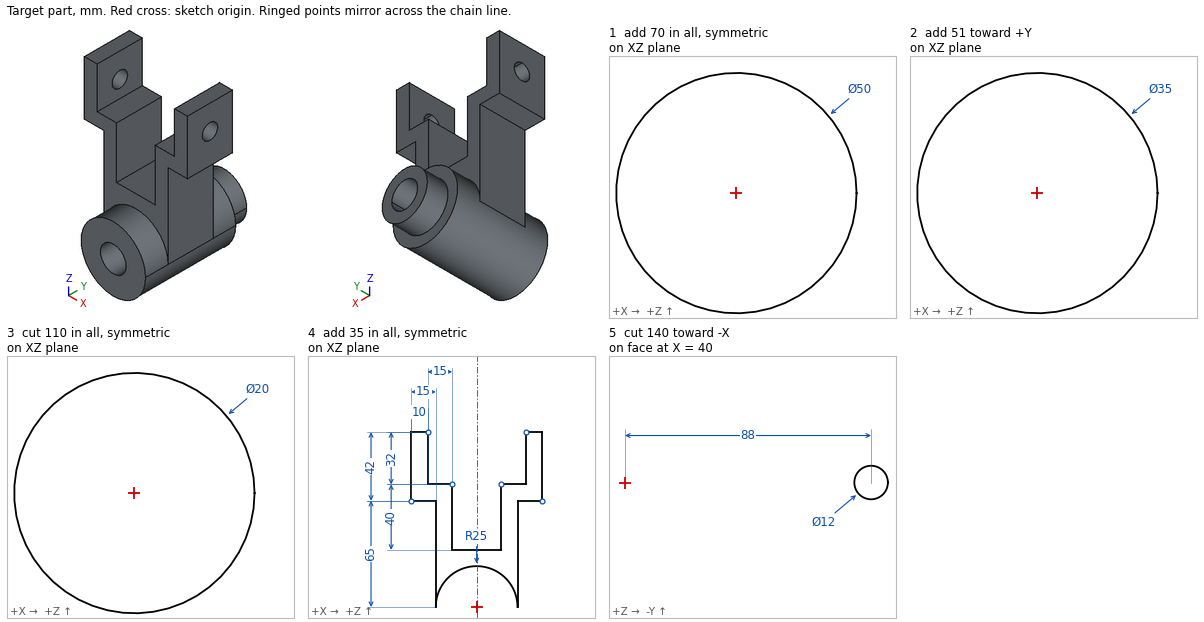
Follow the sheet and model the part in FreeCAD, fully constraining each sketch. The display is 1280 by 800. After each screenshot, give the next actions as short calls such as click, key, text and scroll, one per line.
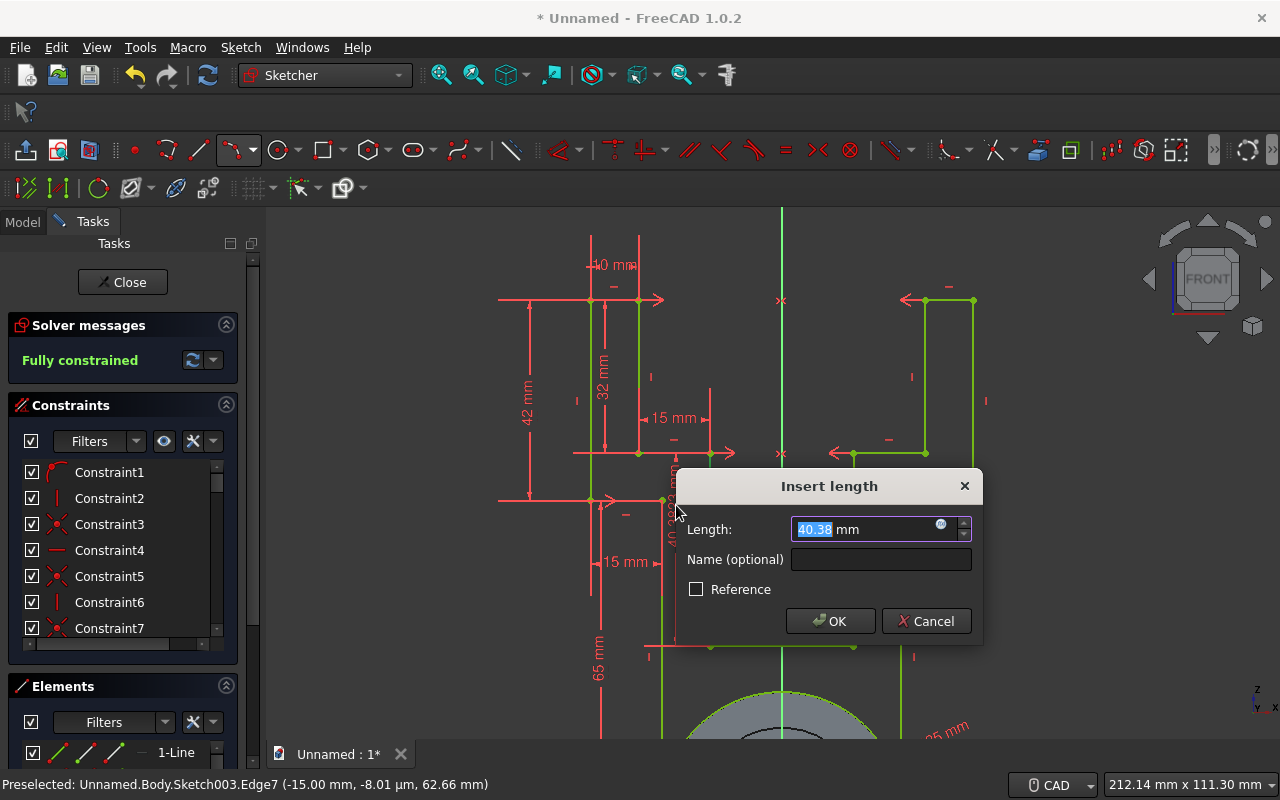
text(40)
key(Return)
key(Escape)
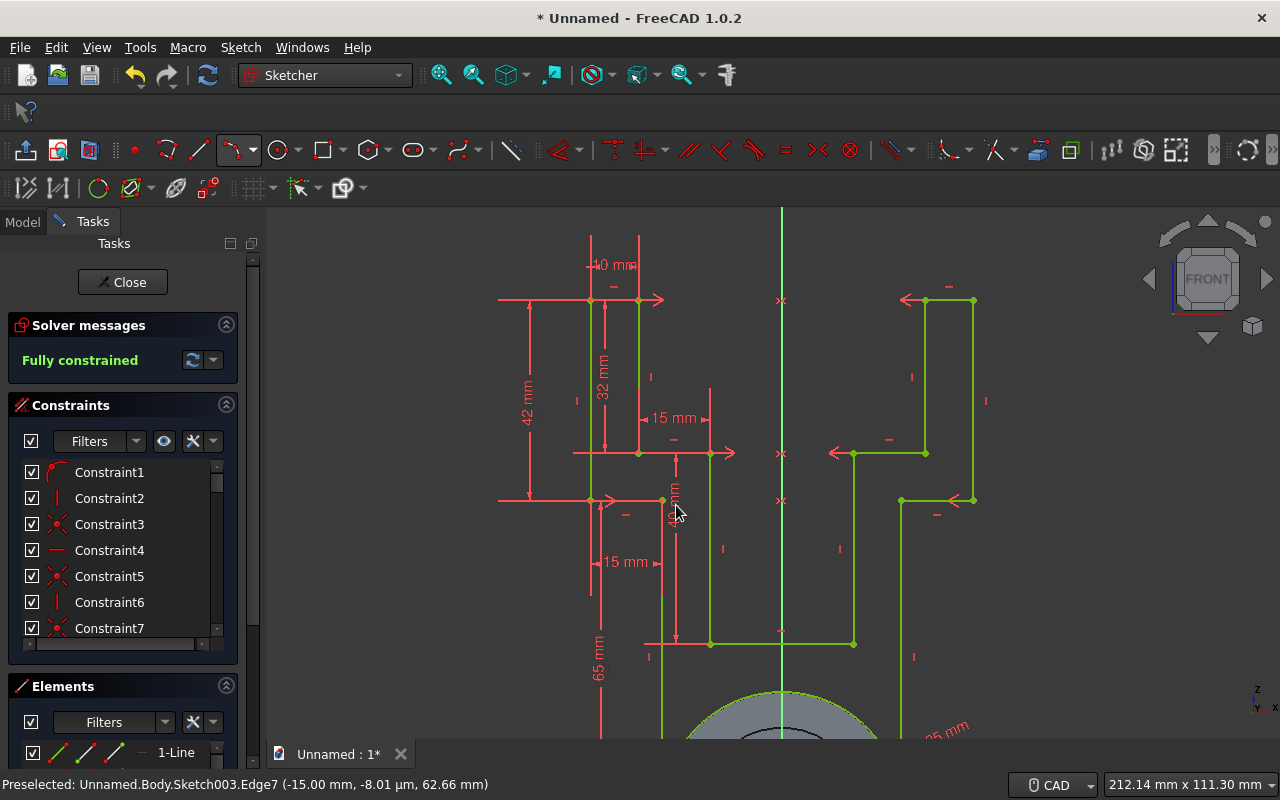
click(123, 282)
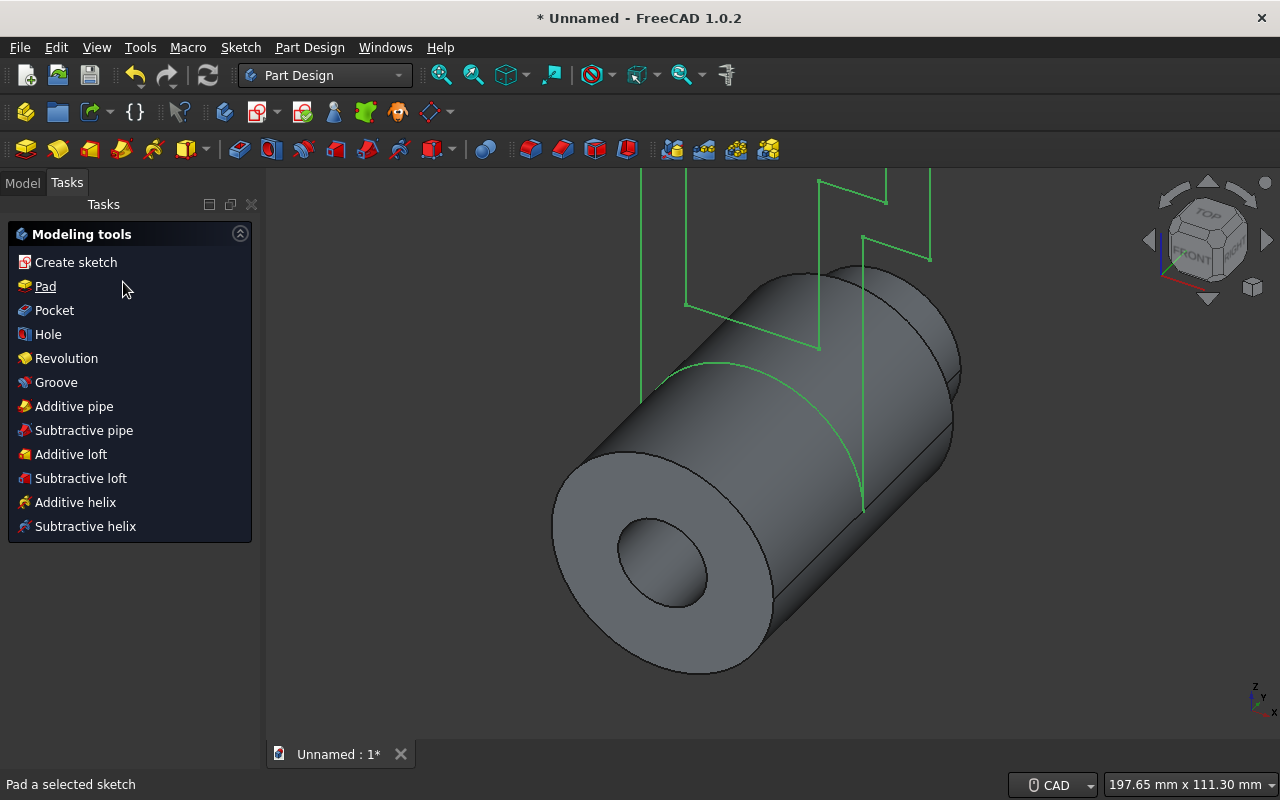
click(26, 150)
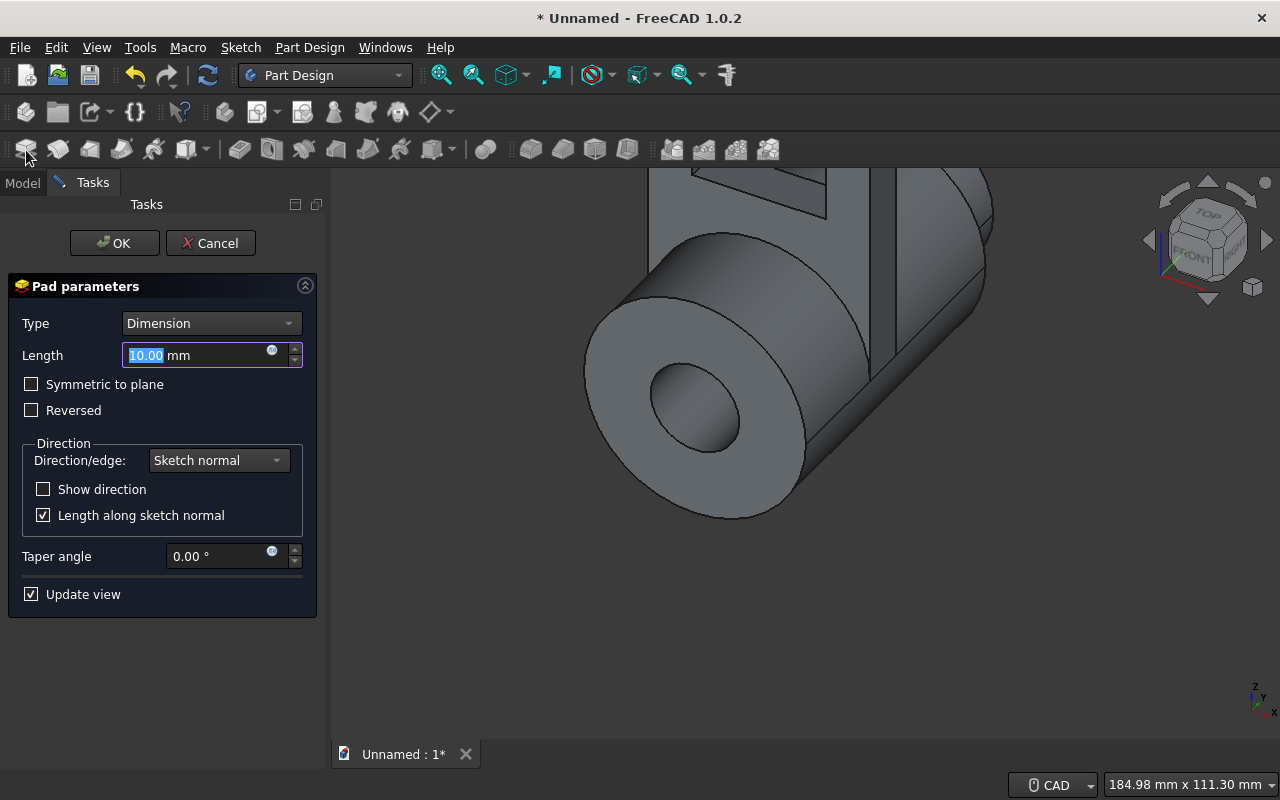
text(35)
key(Tab)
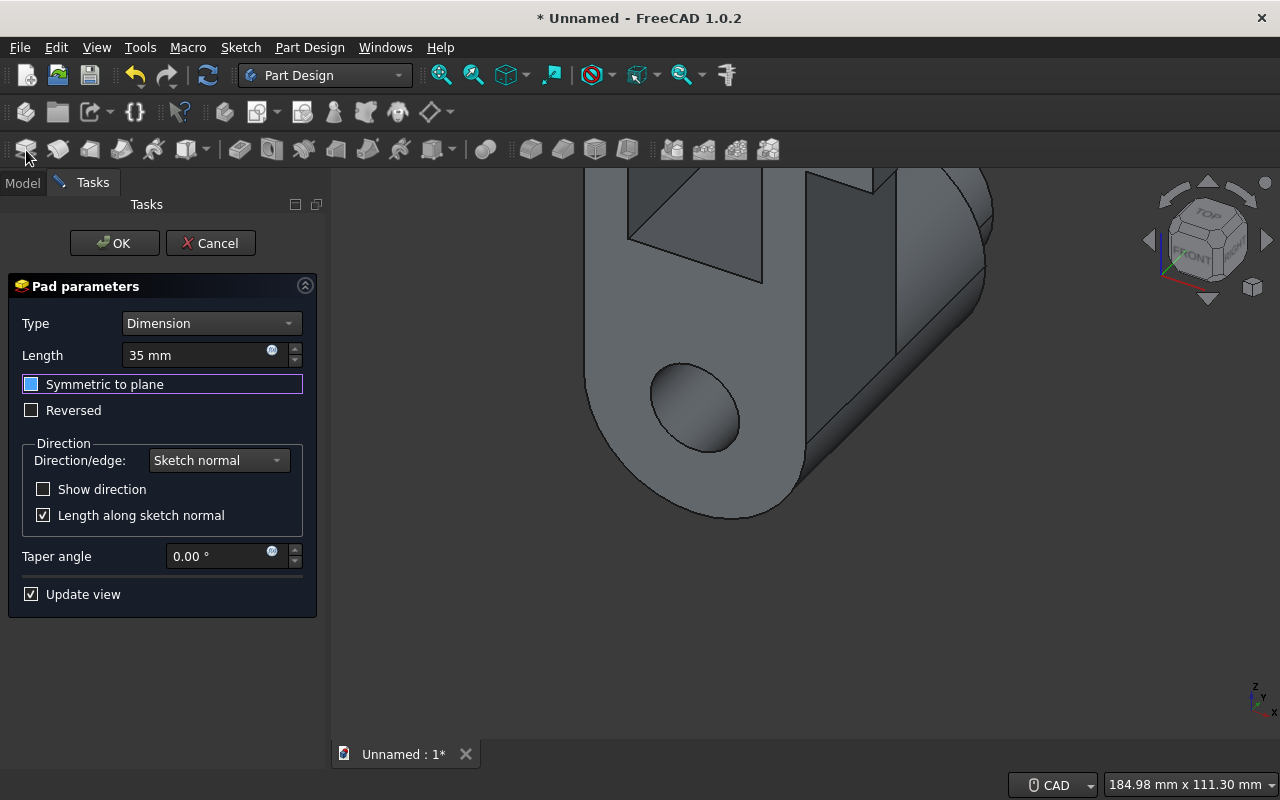
click(30, 384)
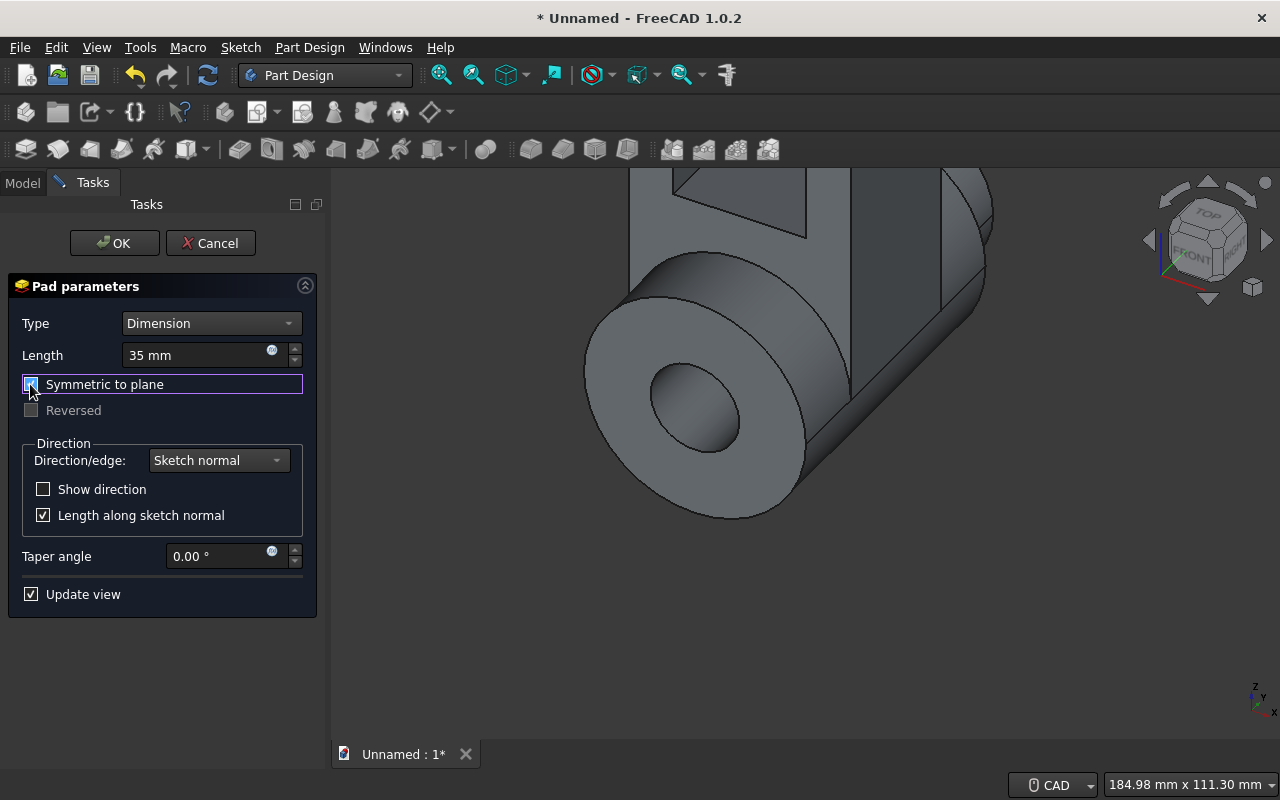
click(115, 243)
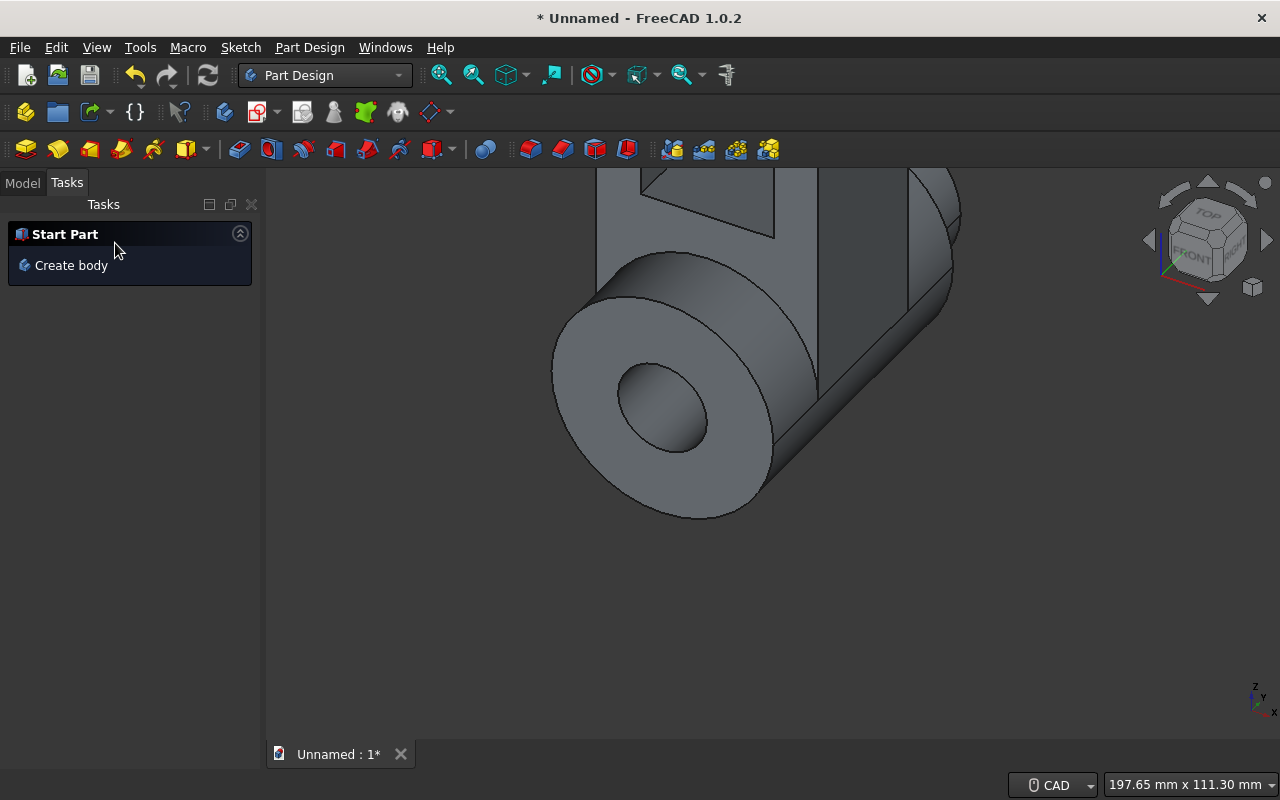
click(442, 76)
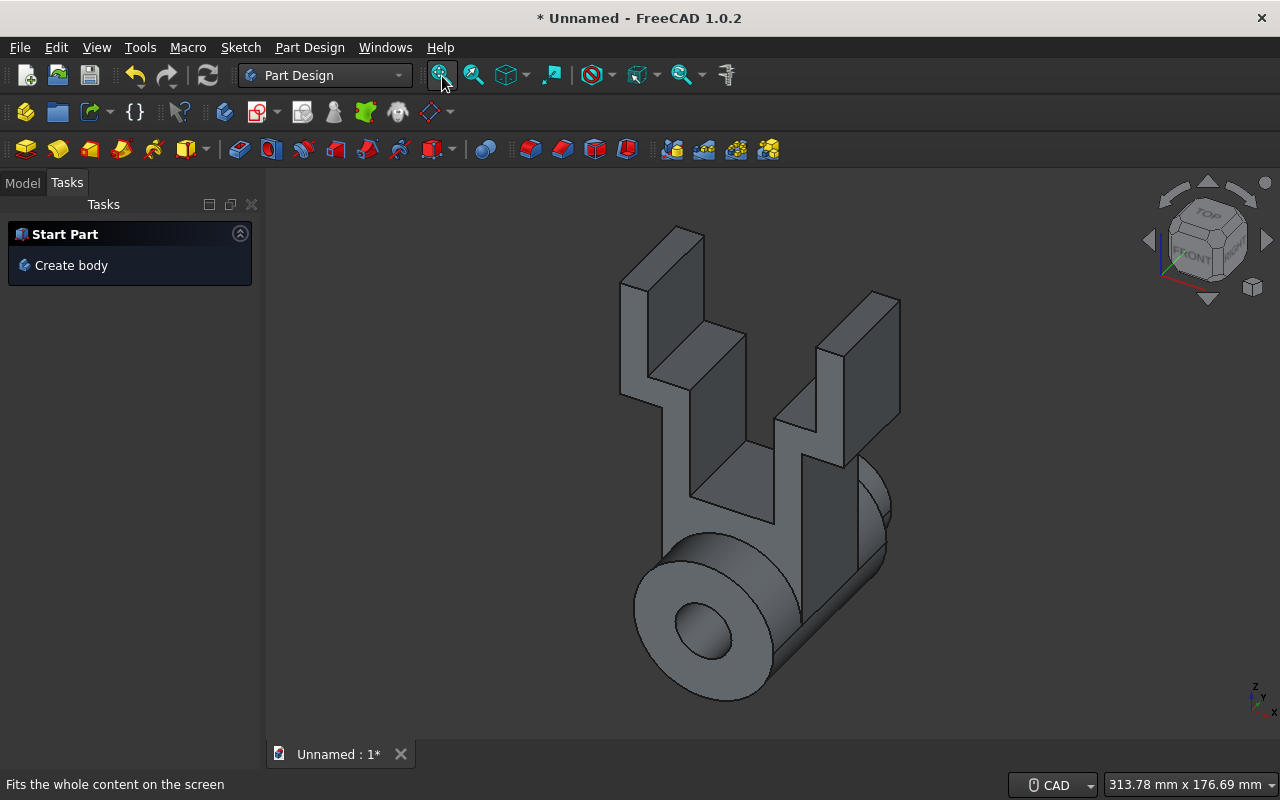
click(872, 383)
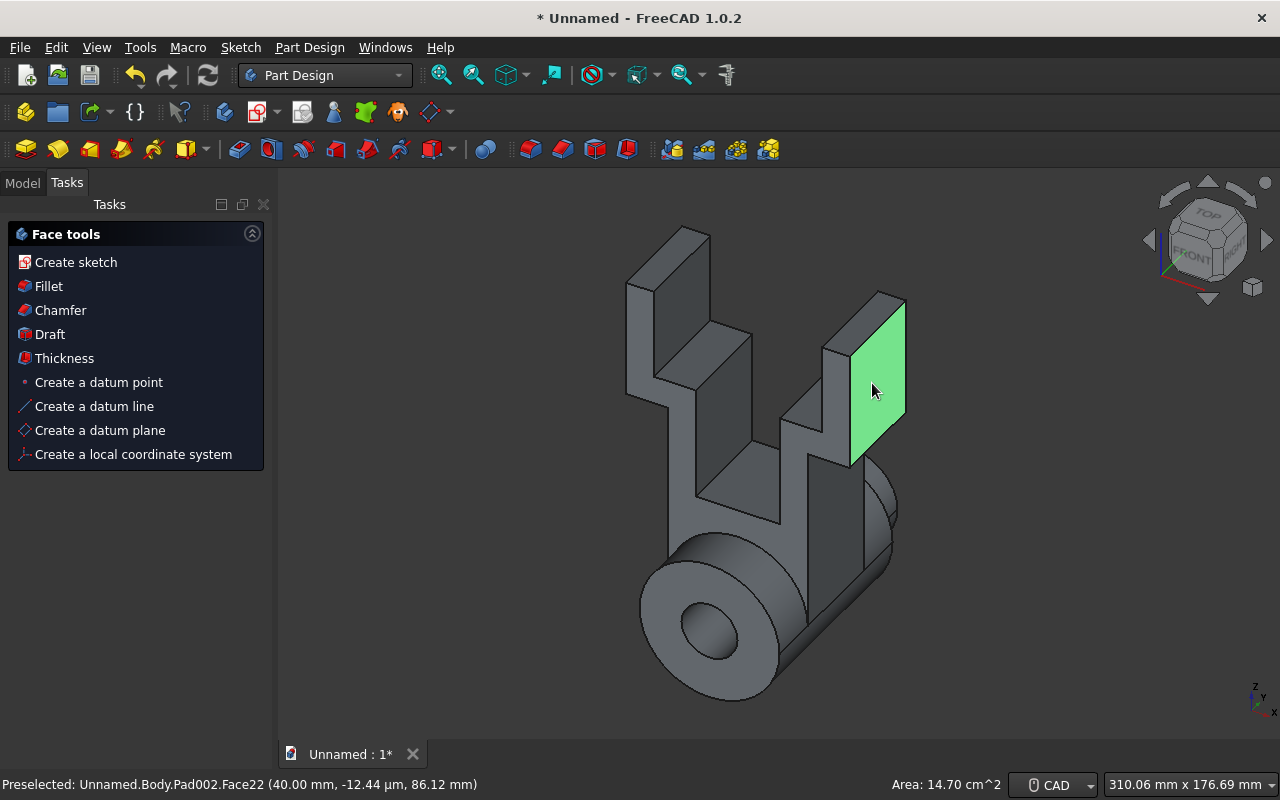
click(258, 112)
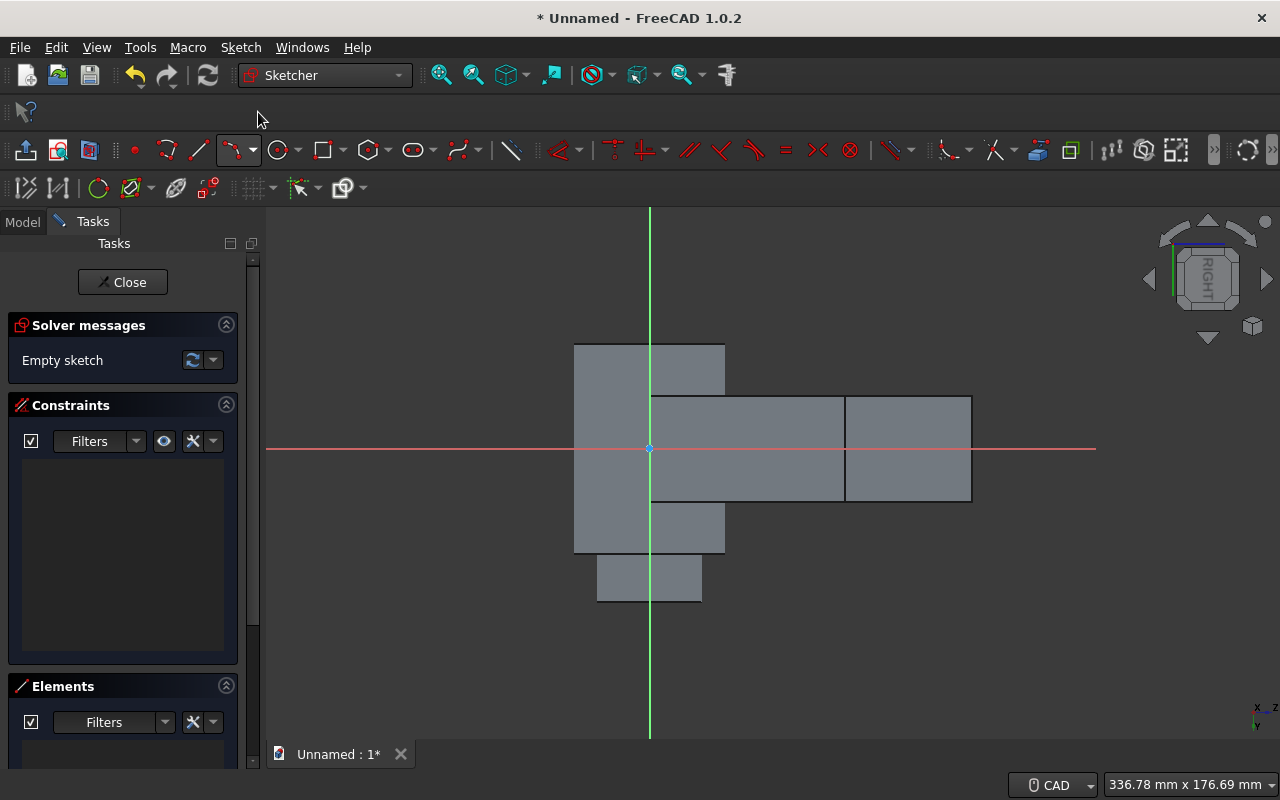
scroll(941, 446, up, 11)